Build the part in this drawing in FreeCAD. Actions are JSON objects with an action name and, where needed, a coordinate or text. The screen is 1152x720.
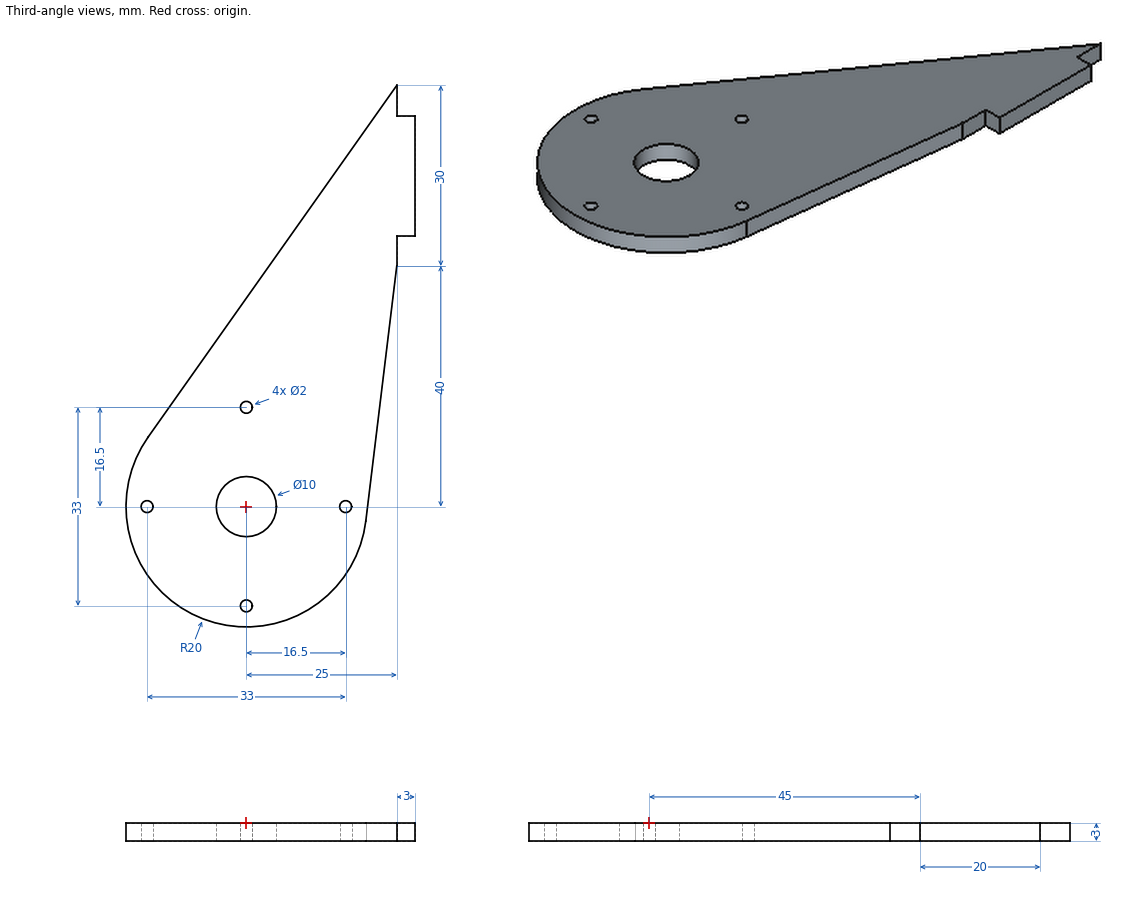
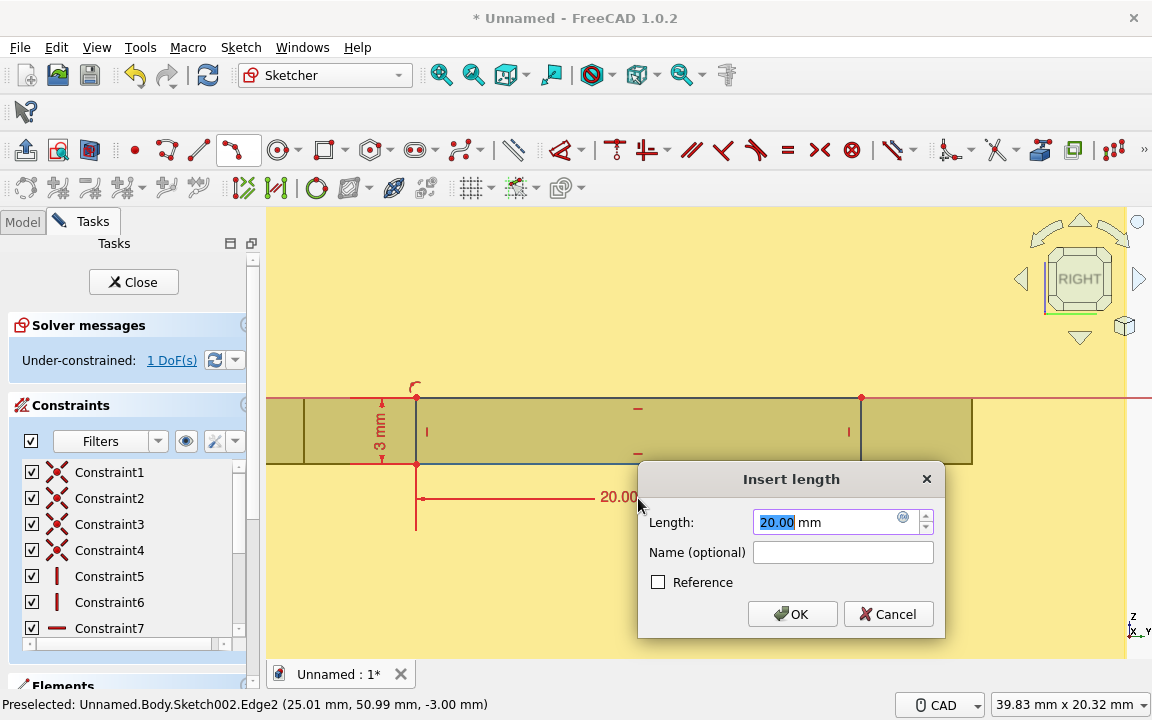
{"action": "type", "text": "20"}
{"action": "key", "text": "Return"}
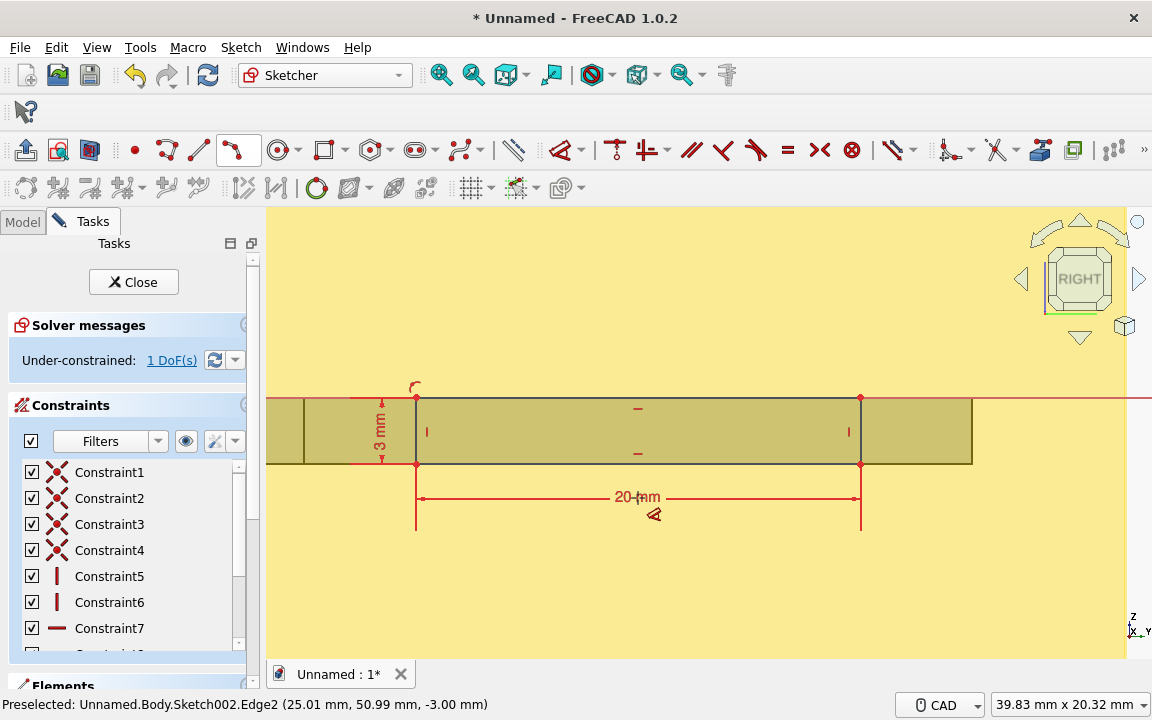
{"action": "left_click", "coordinate": [416, 398]}
{"action": "left_click", "coordinate": [355, 364]}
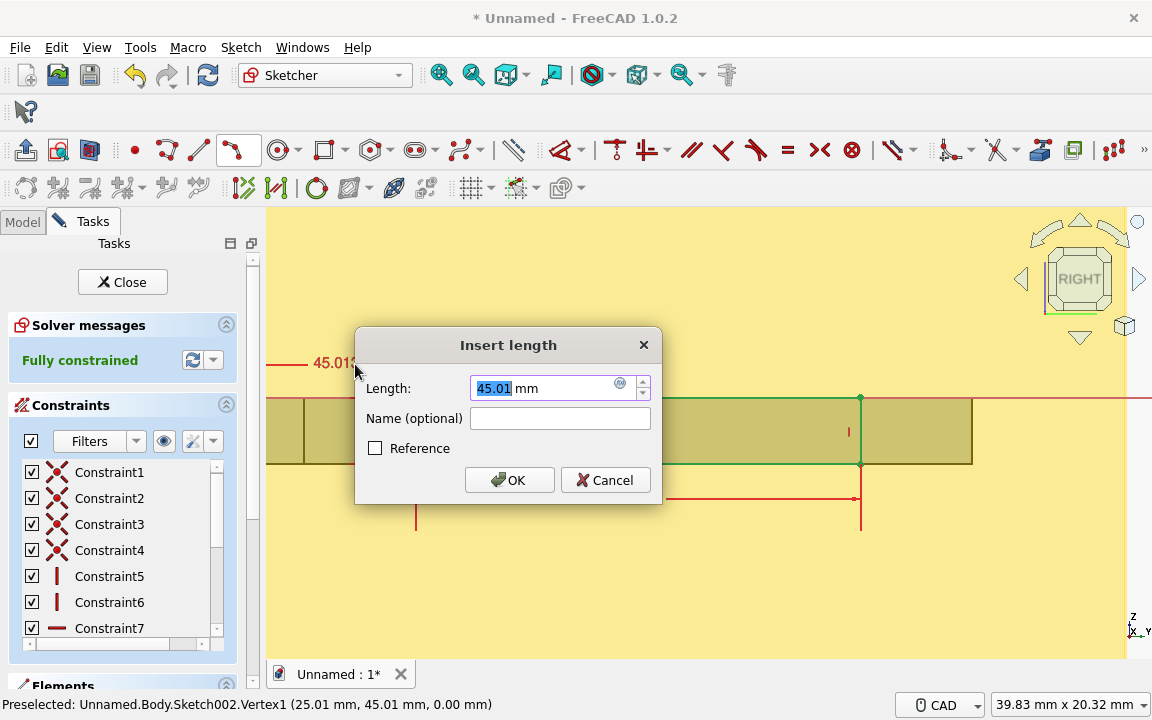
{"action": "type", "text": "45"}
{"action": "key", "text": "Return"}
{"action": "key", "text": "Escape"}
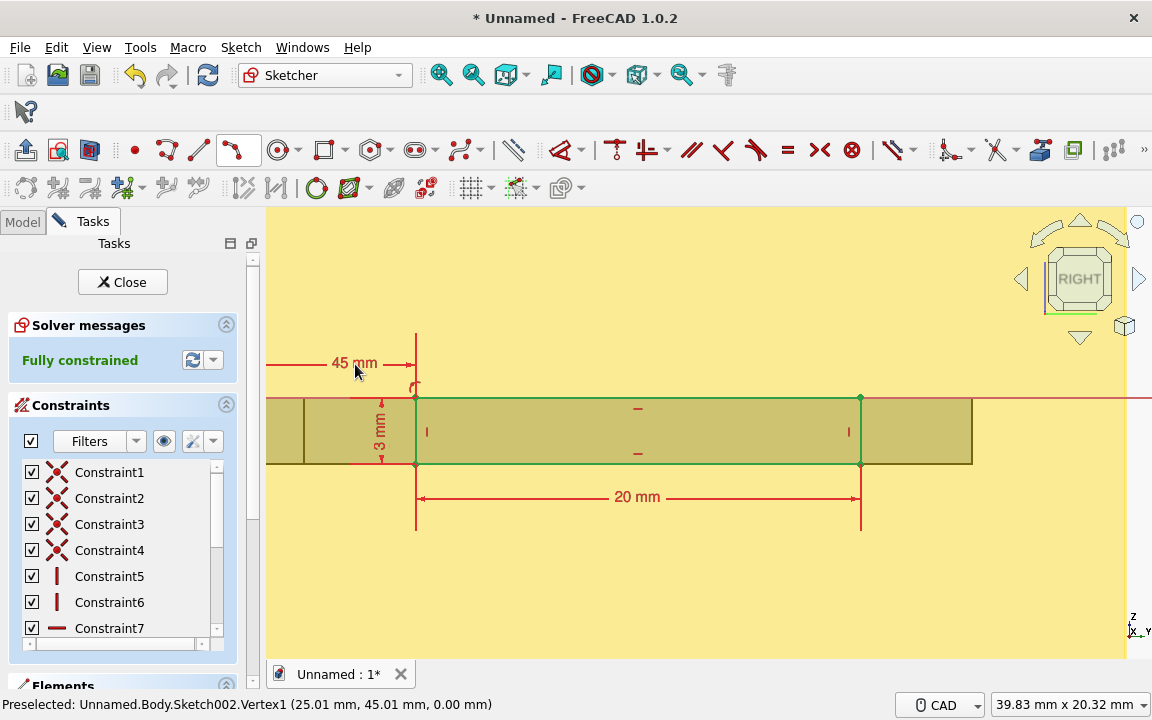
{"action": "left_click", "coordinate": [123, 282]}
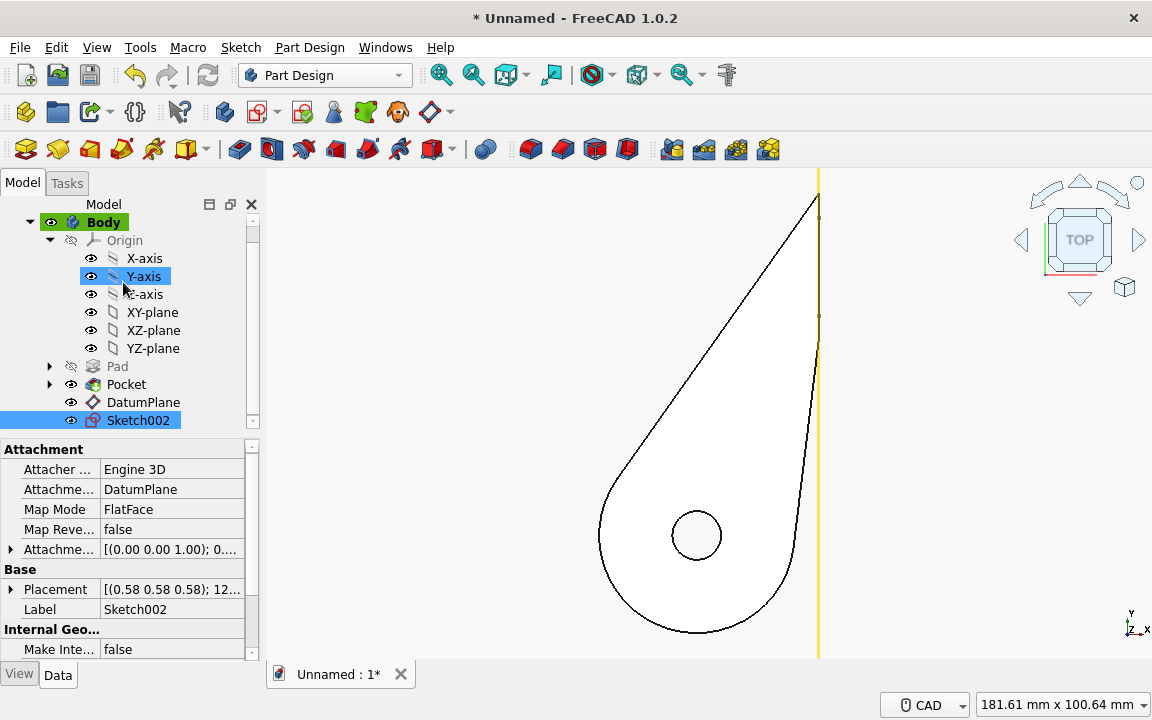
{"action": "left_click", "coordinate": [26, 150]}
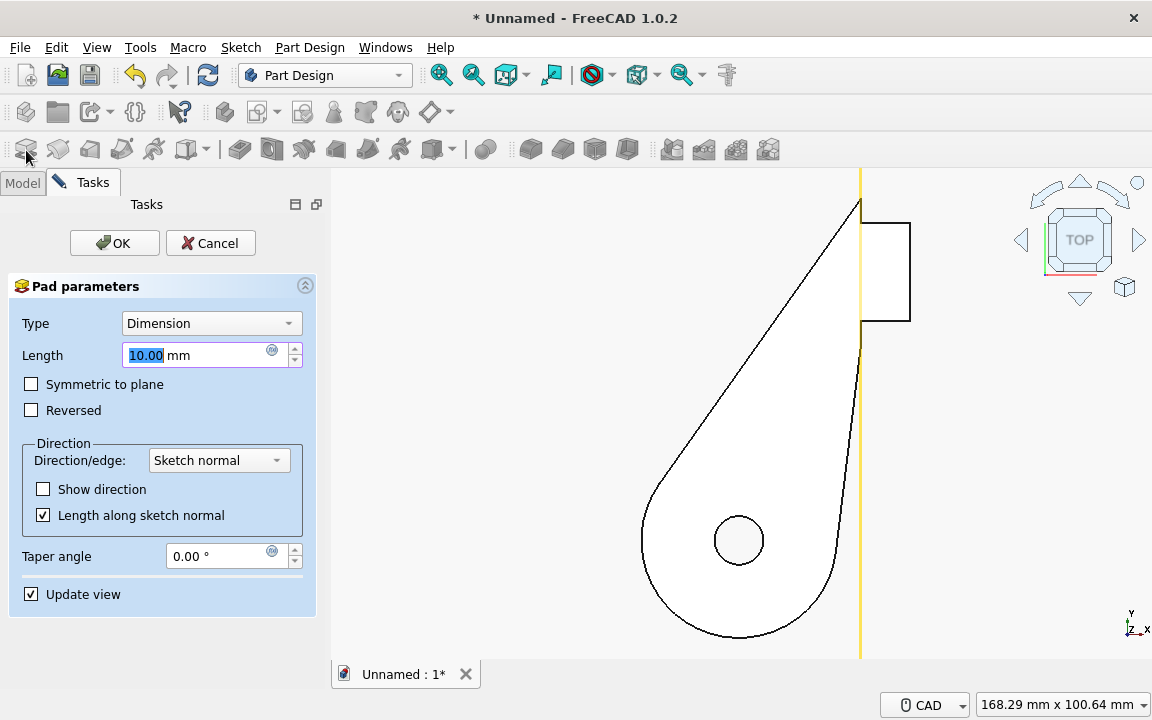
{"action": "type", "text": "3"}
{"action": "key", "text": "Tab"}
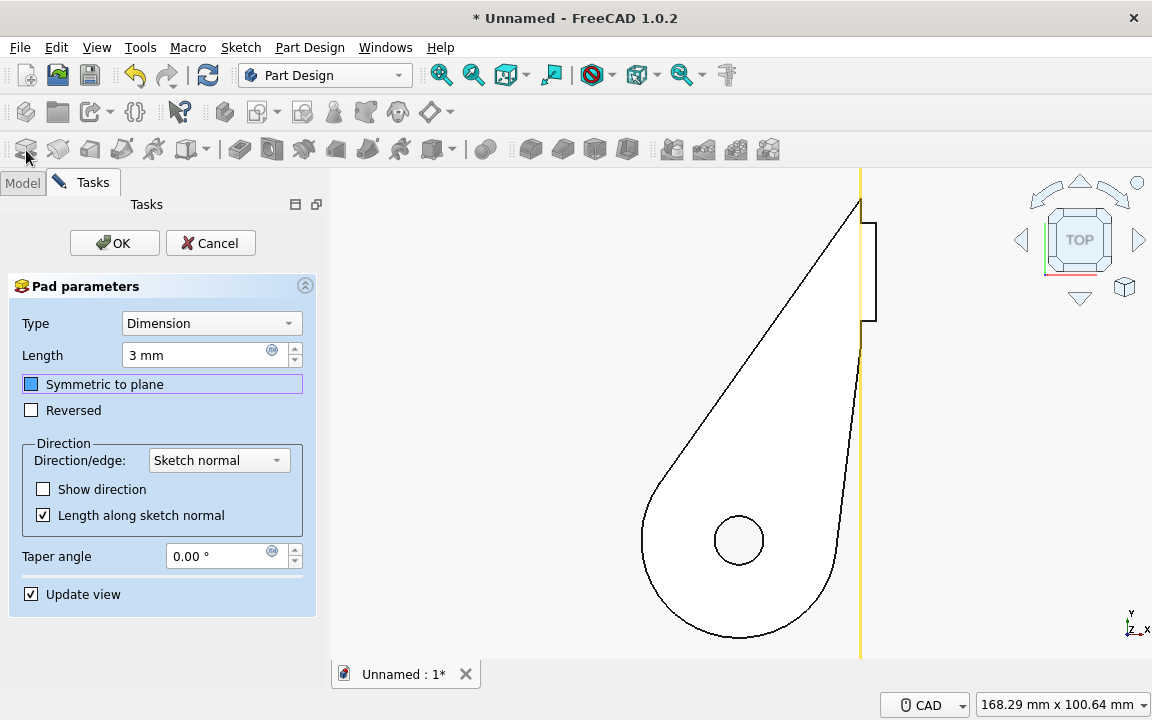
{"action": "left_click", "coordinate": [115, 243]}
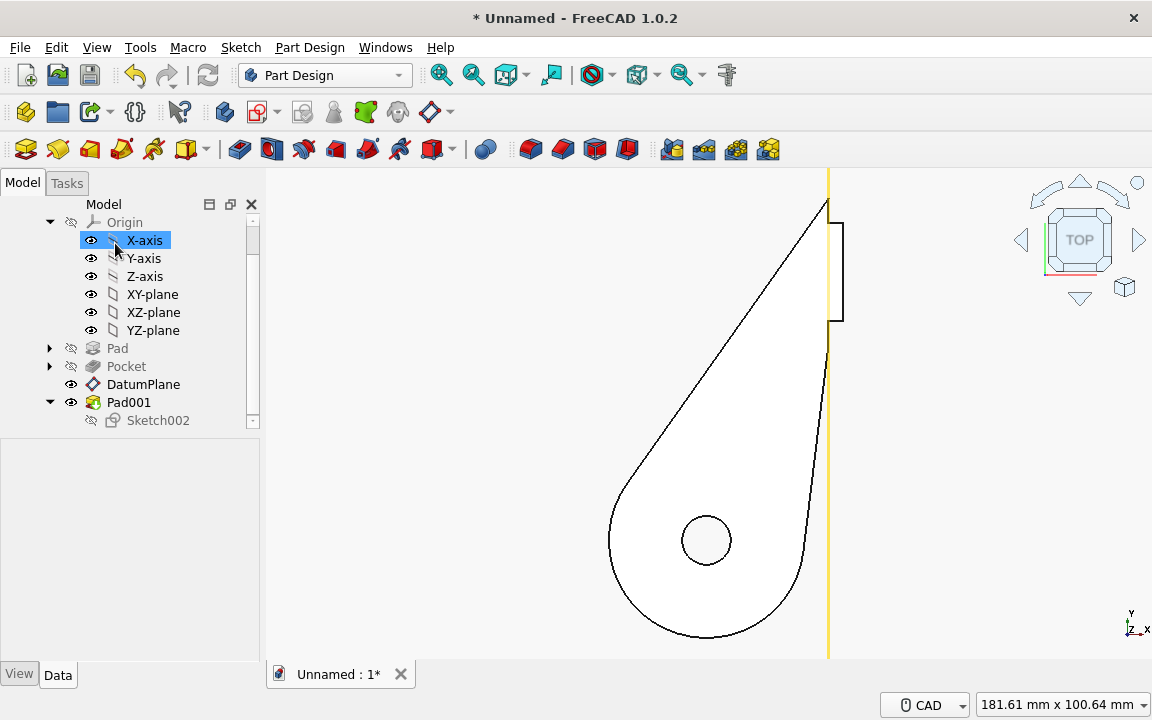
{"action": "left_click", "coordinate": [116, 384]}
{"action": "key", "text": "space"}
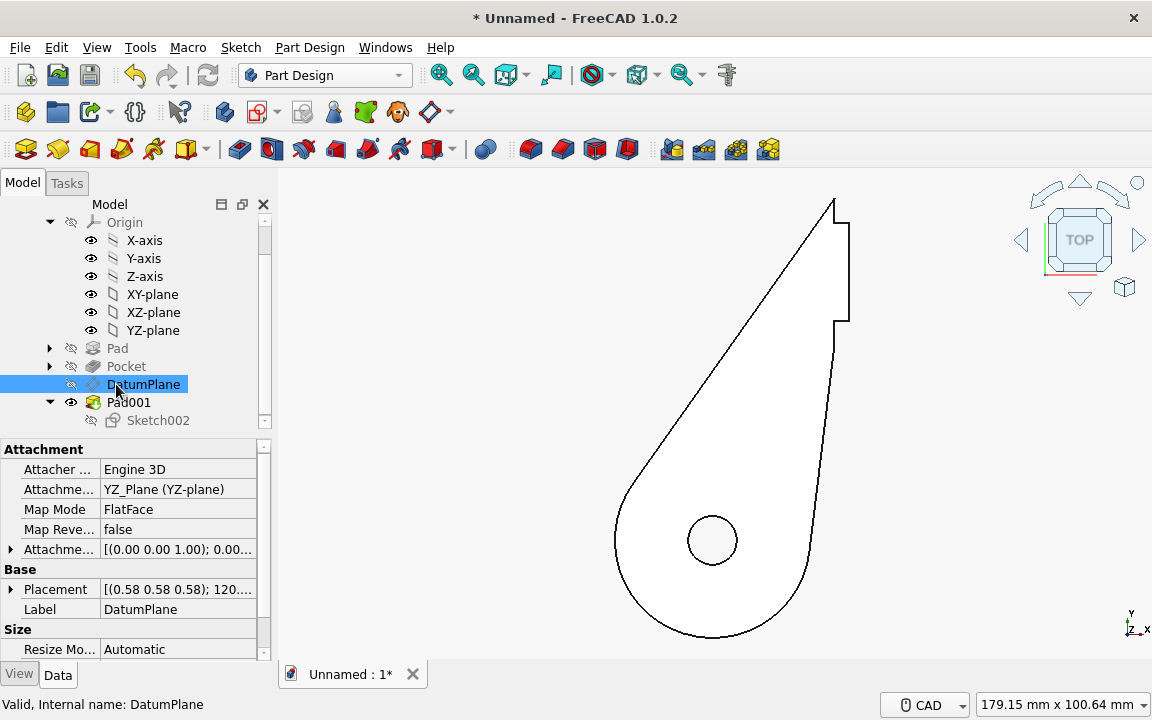
{"action": "left_click", "coordinate": [318, 619]}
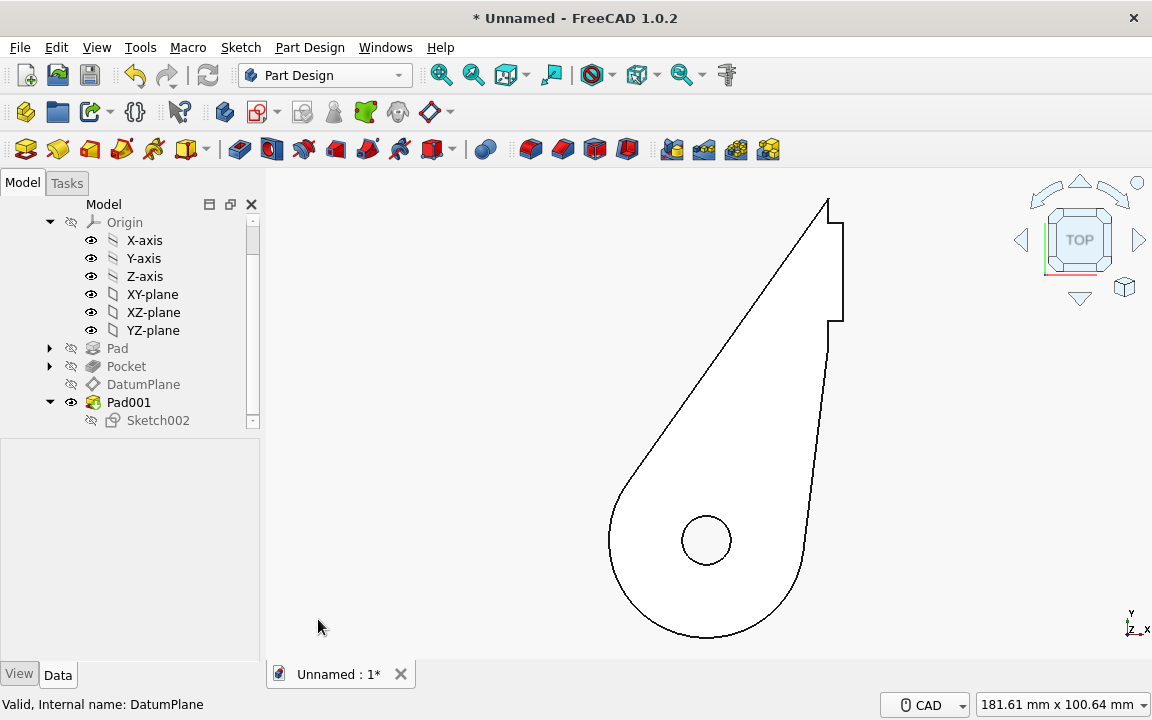
{"action": "left_click", "coordinate": [258, 112]}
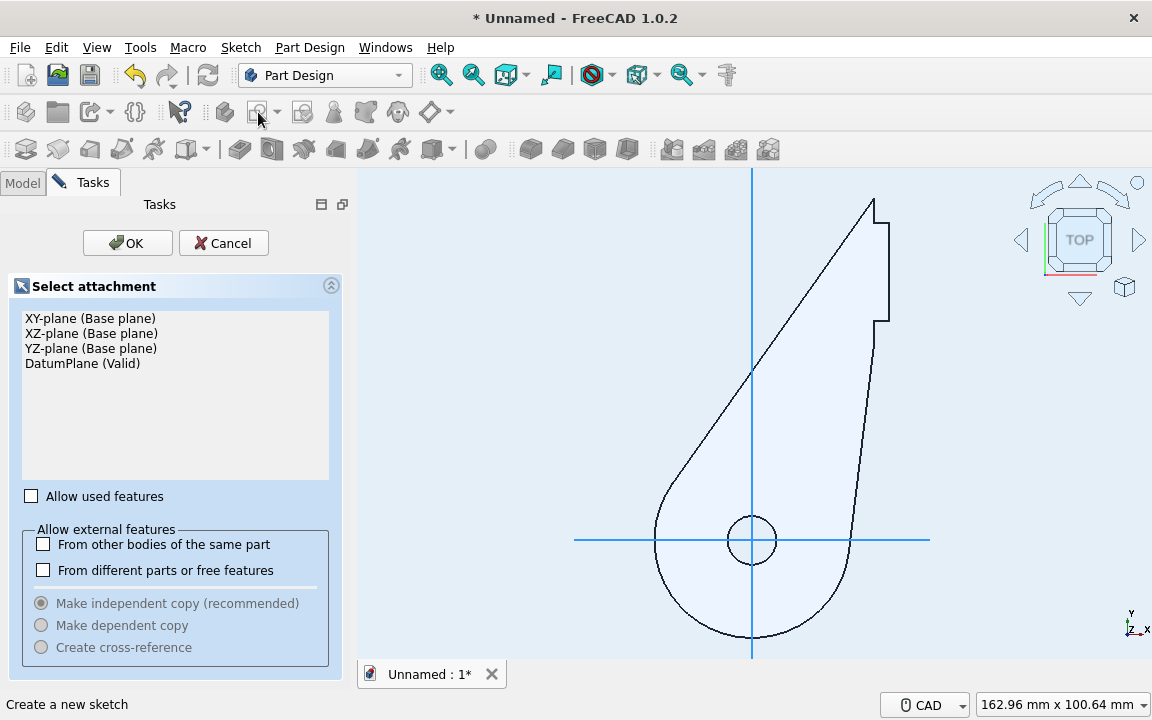
{"action": "left_click", "coordinate": [82, 318]}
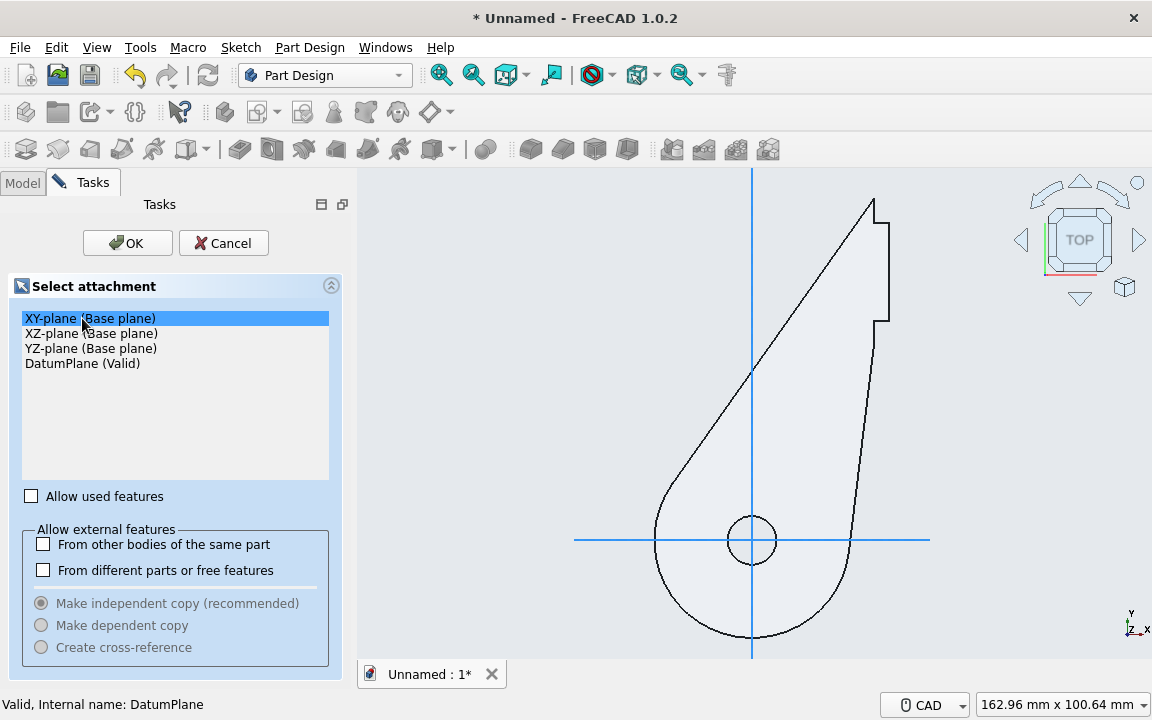
{"action": "left_click", "coordinate": [128, 243]}